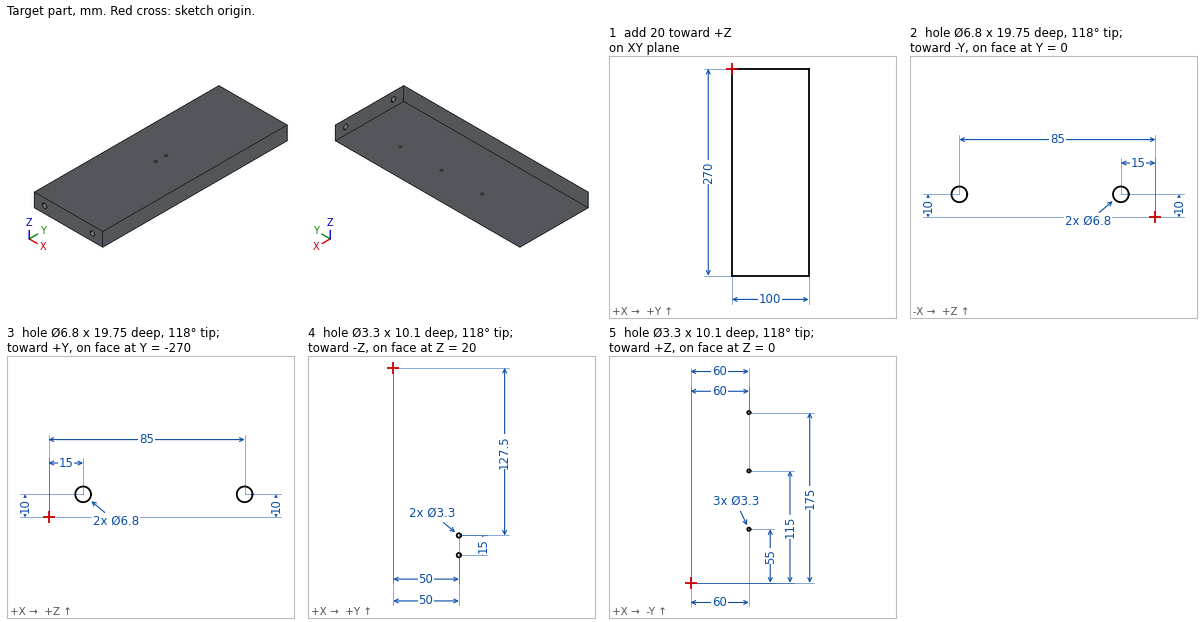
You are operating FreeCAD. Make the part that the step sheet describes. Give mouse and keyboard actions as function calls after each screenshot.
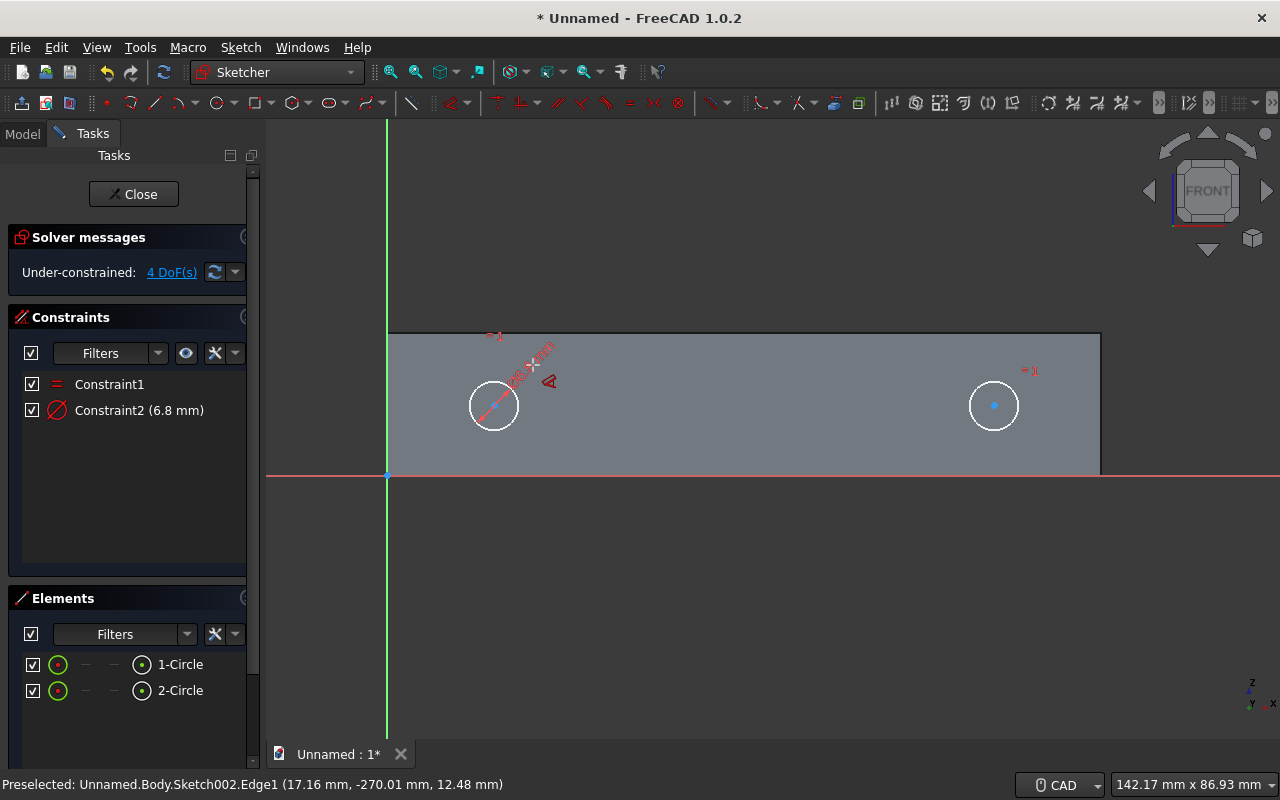
click(494, 406)
click(441, 510)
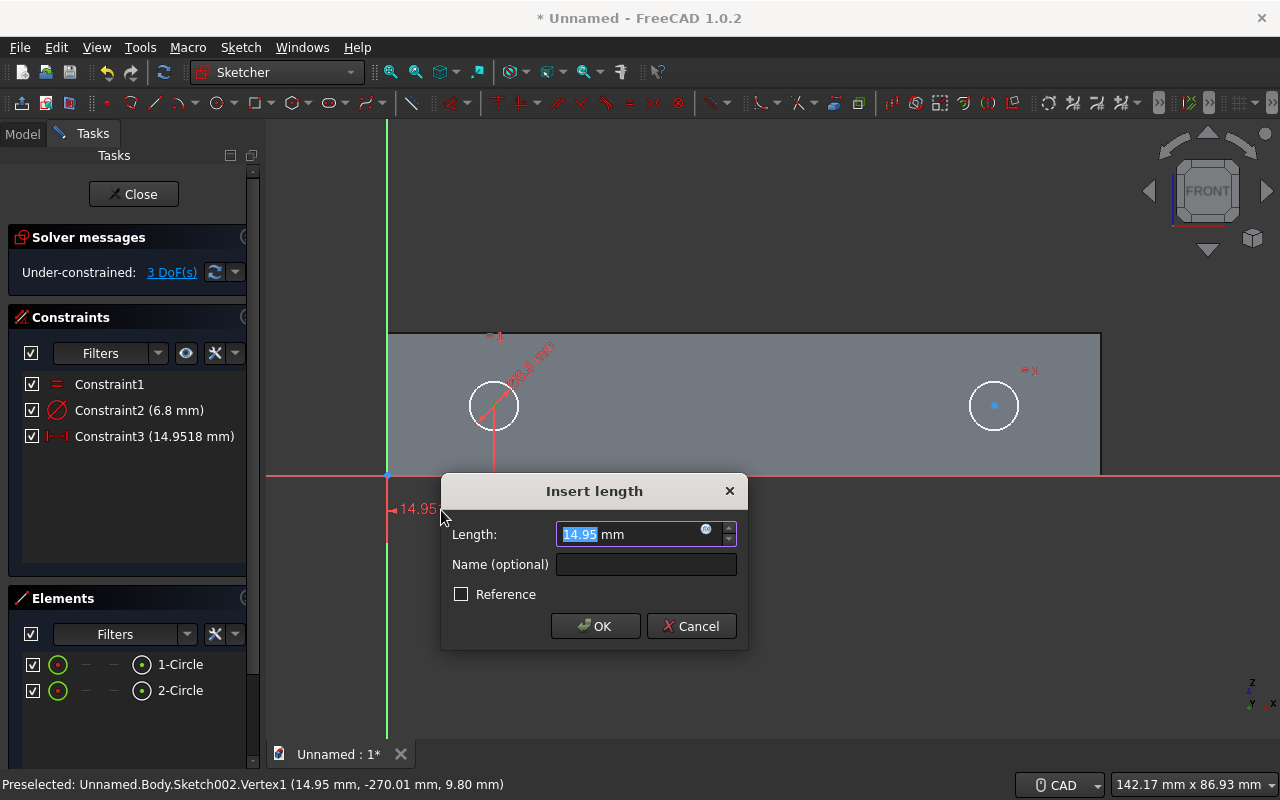
text(15)
key(Return)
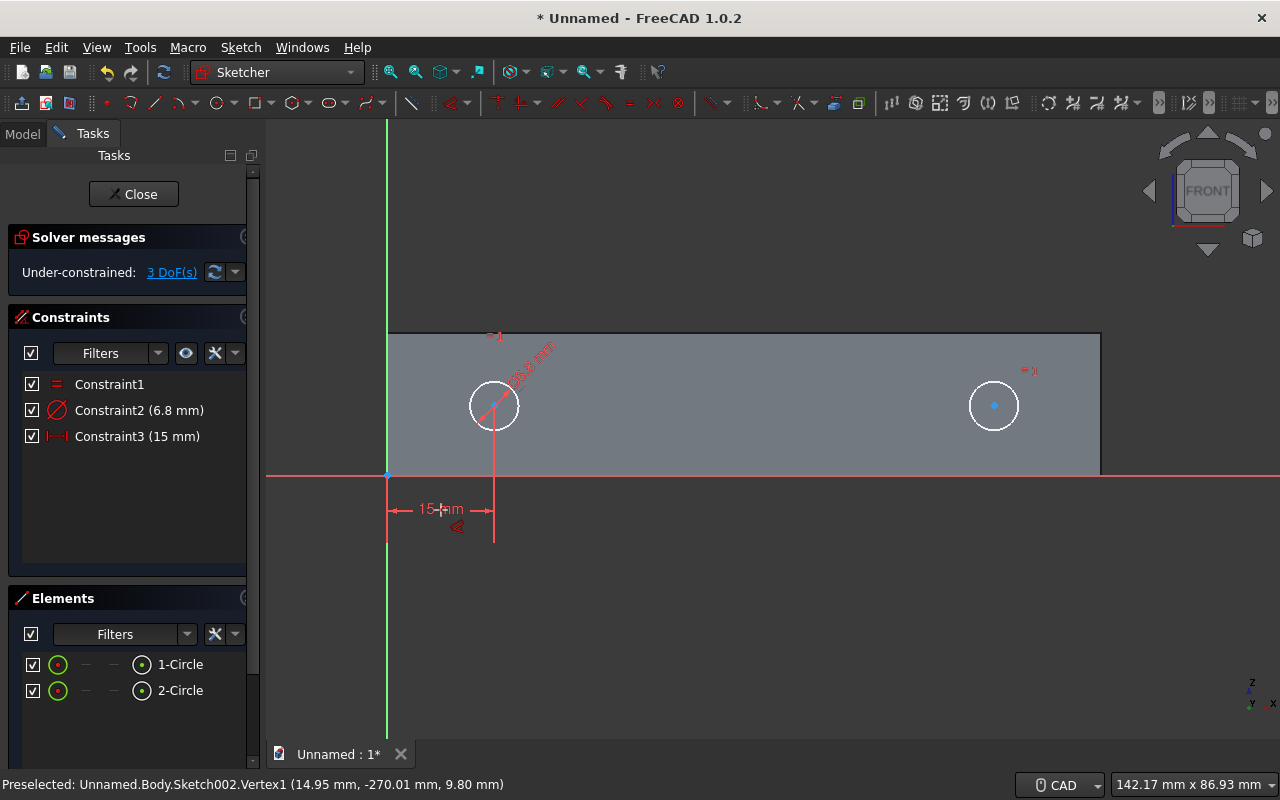
click(494, 406)
click(353, 441)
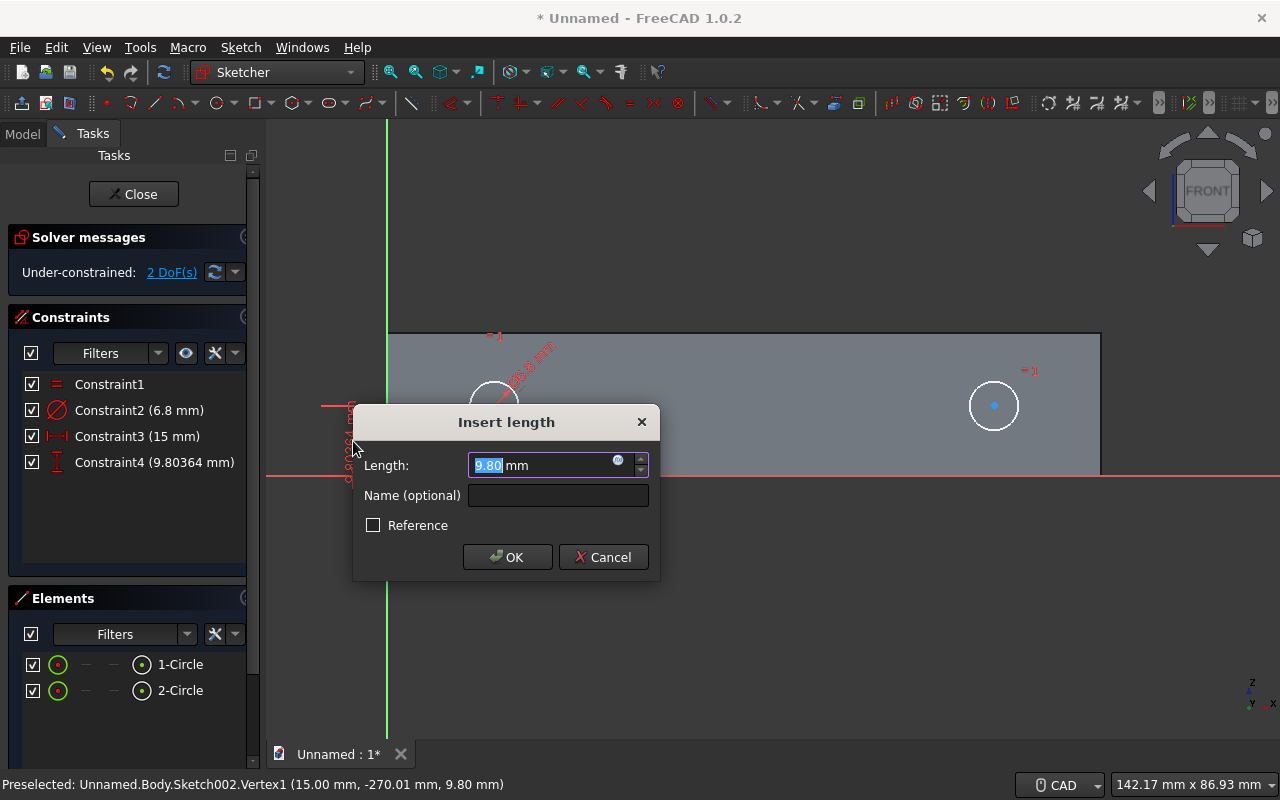
text(10)
key(Return)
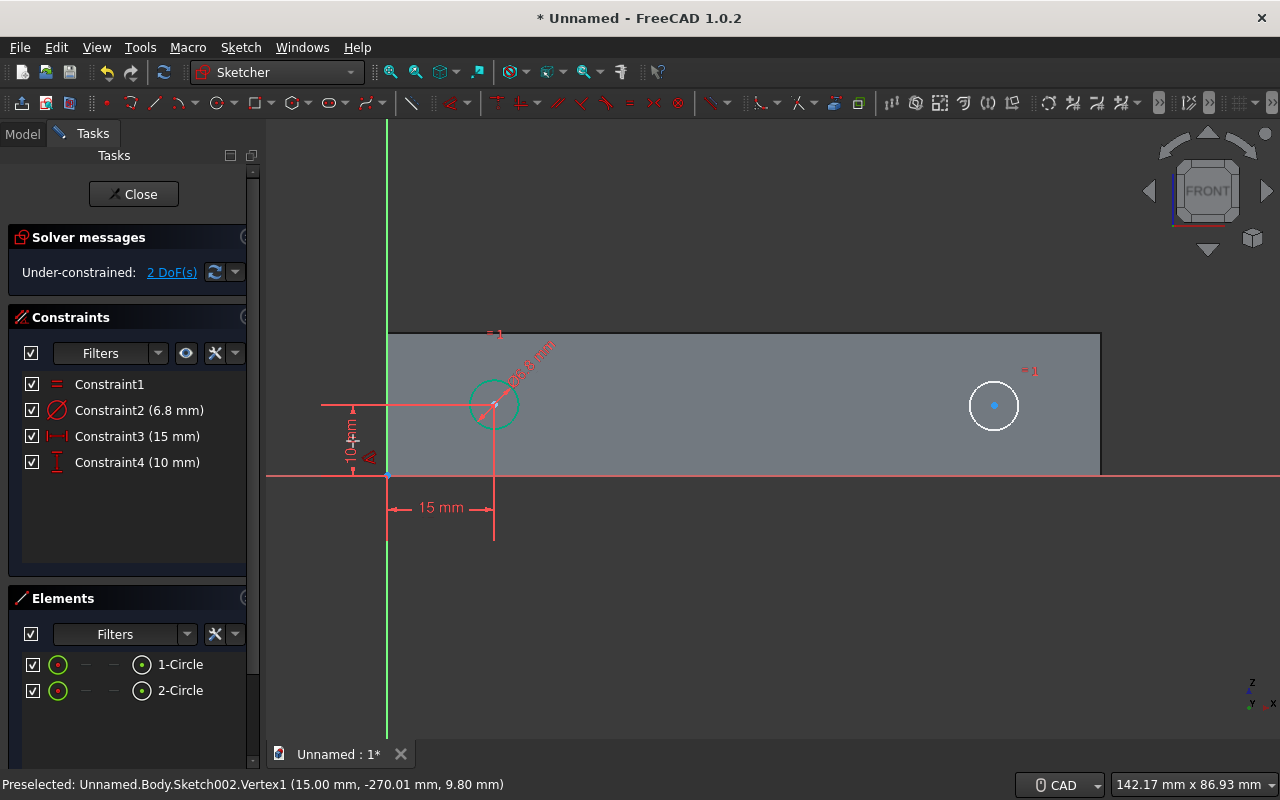
click(994, 406)
click(691, 510)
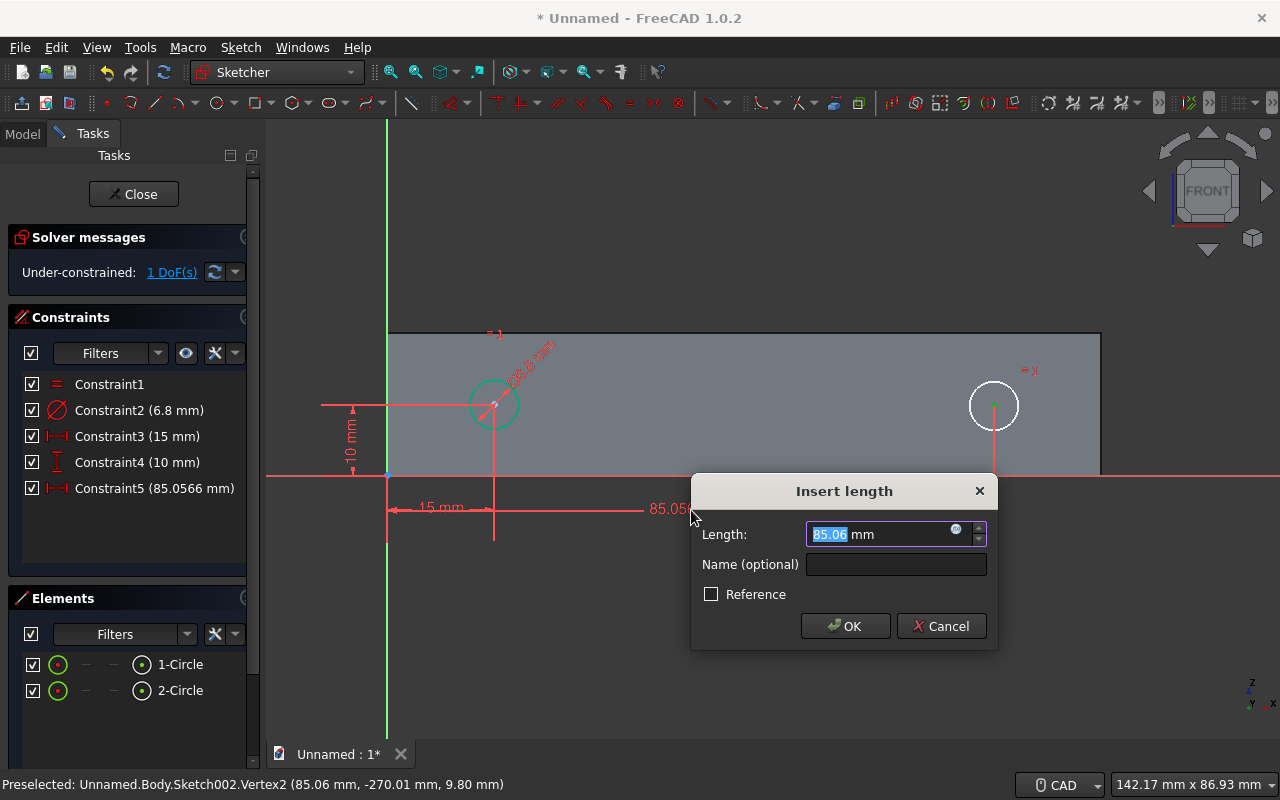
text(85)
key(Return)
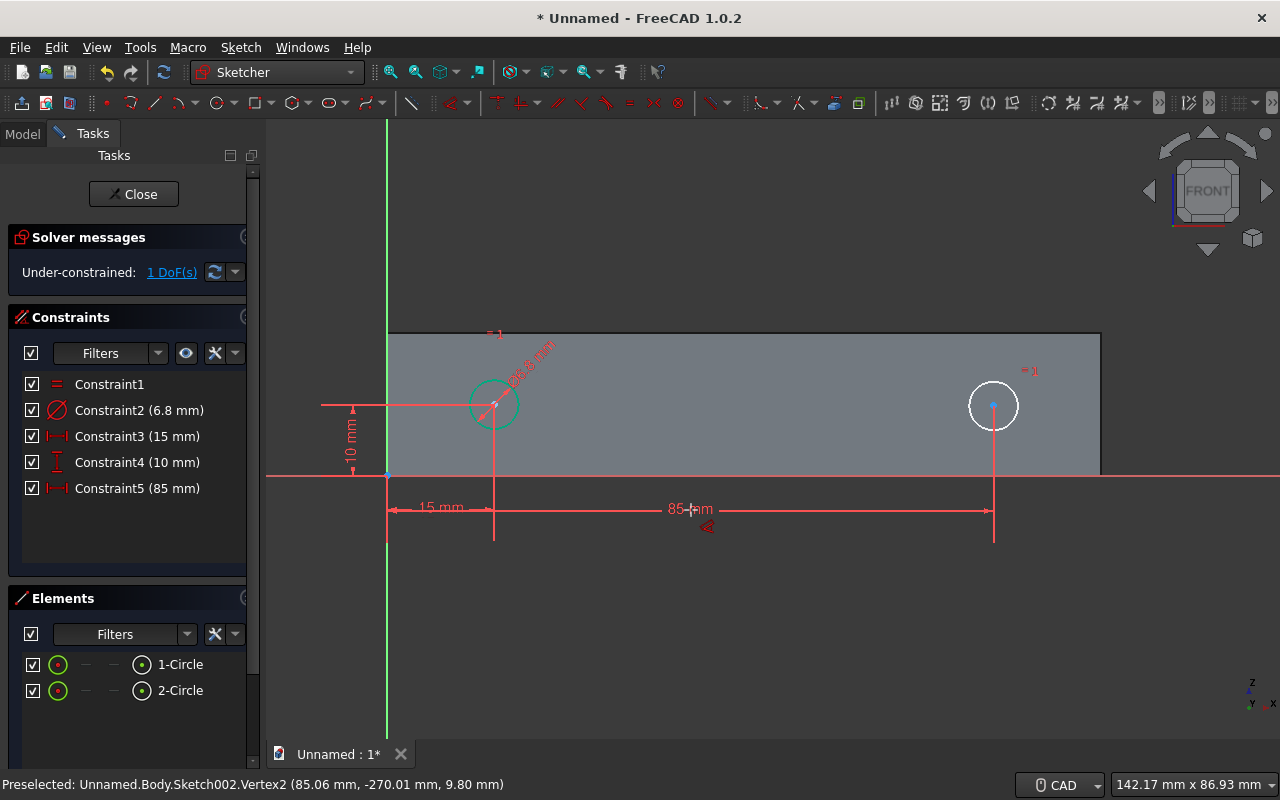
click(994, 406)
click(353, 416)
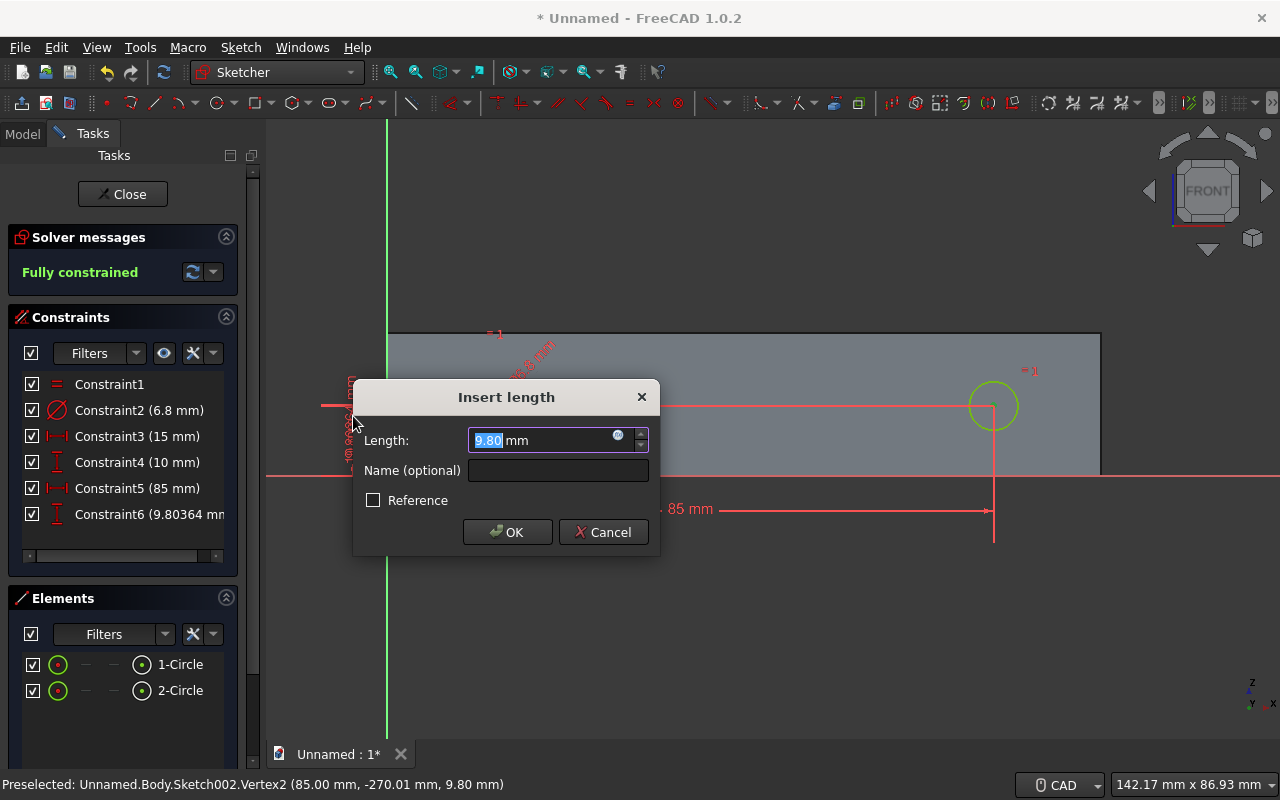
text(10)
key(Return)
key(Escape)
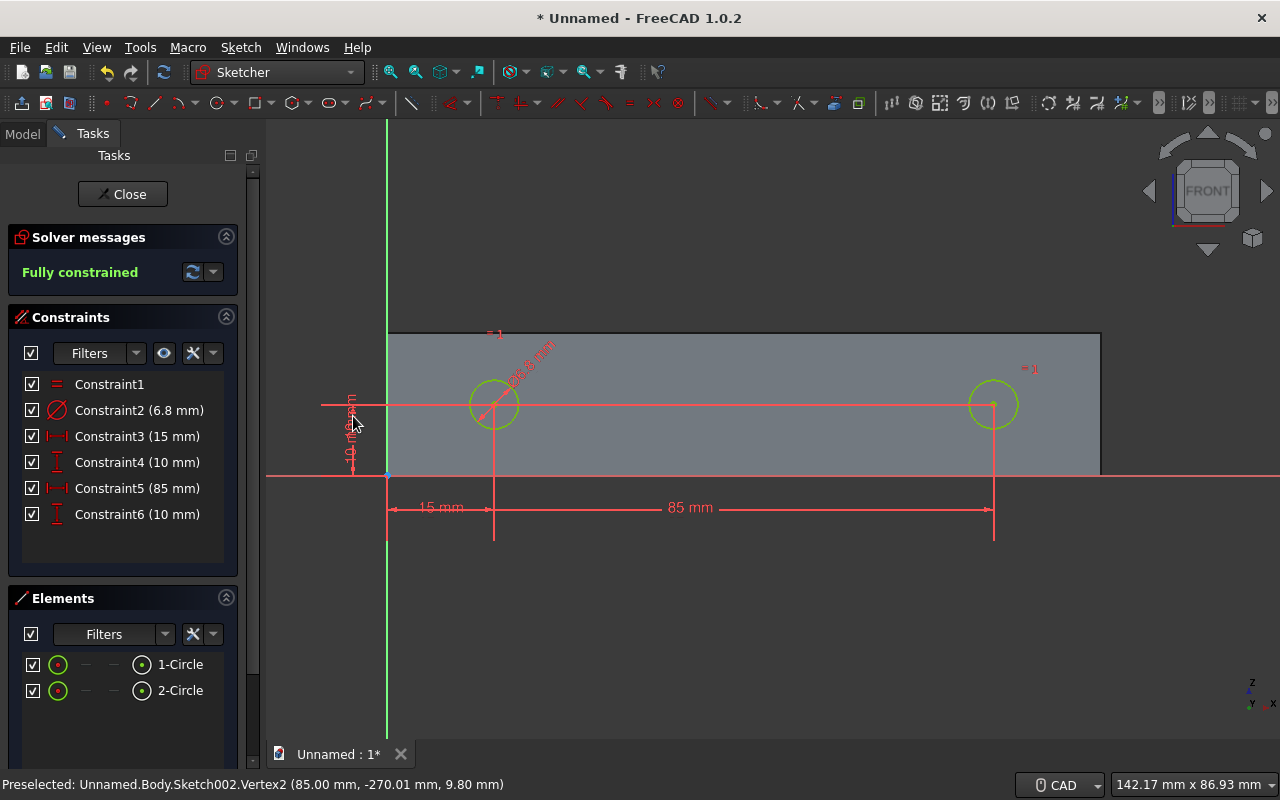
click(123, 194)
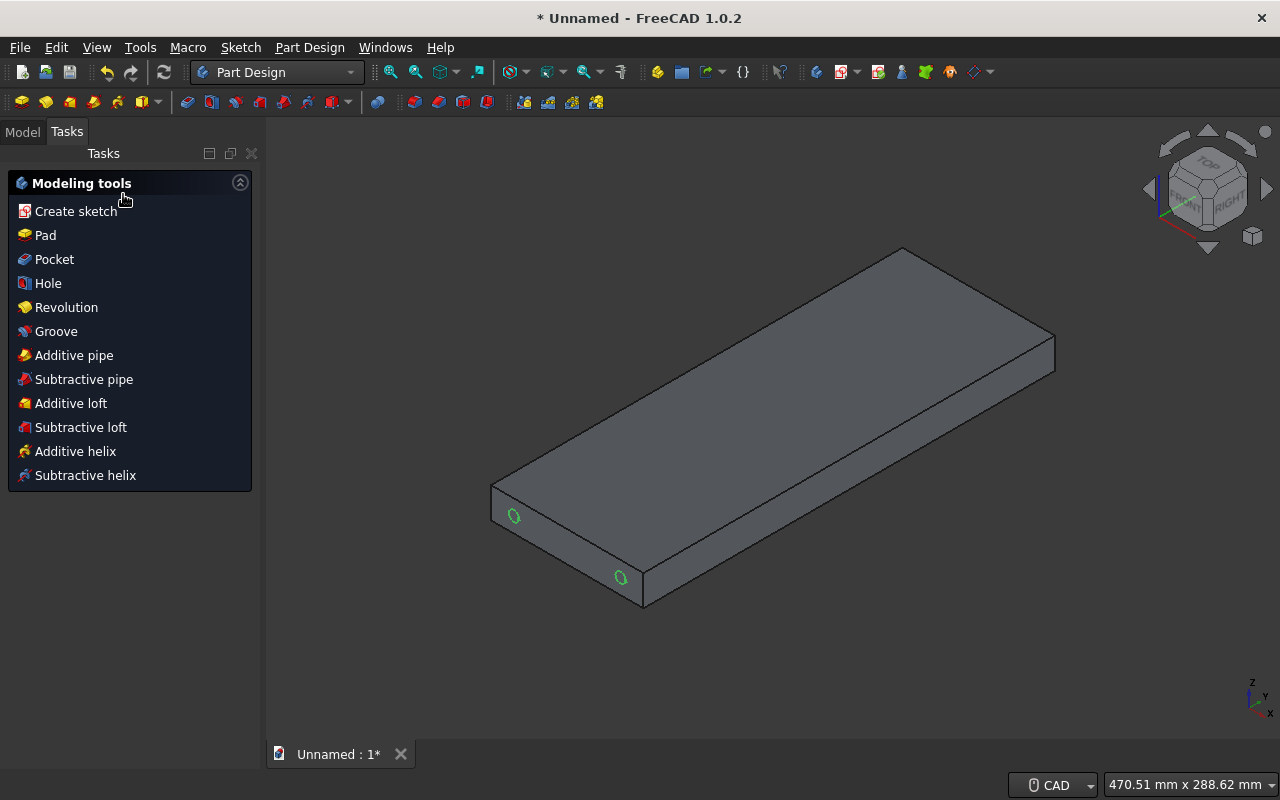
click(212, 102)